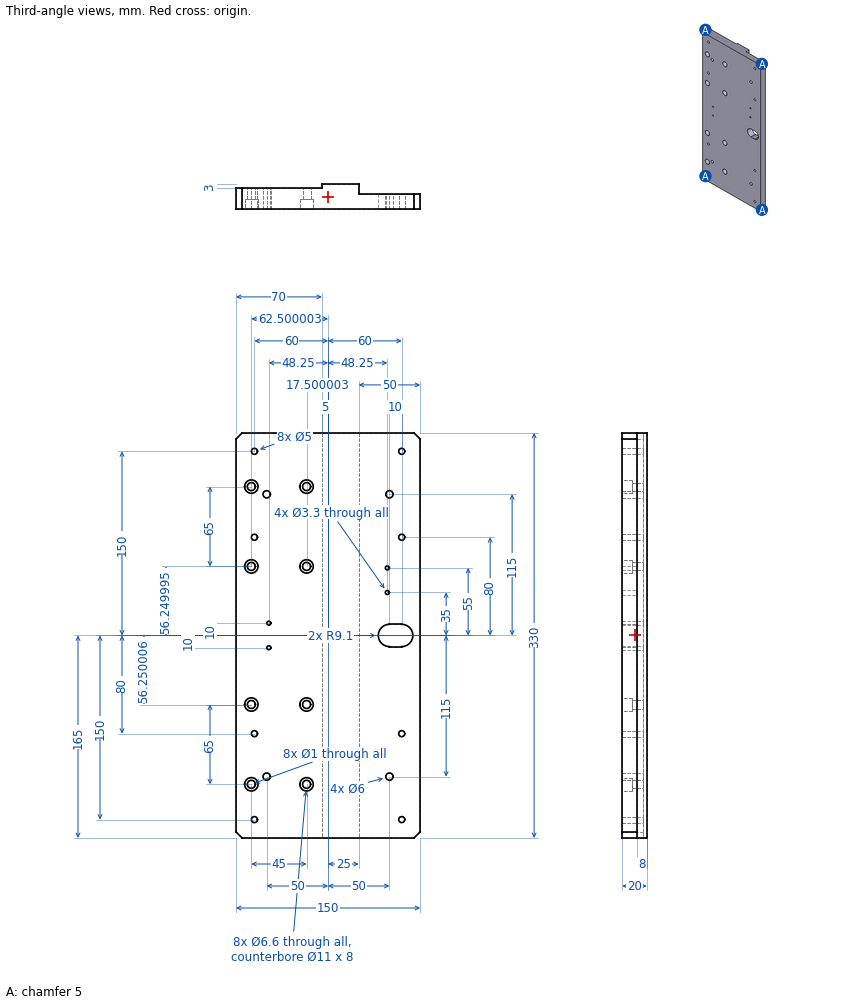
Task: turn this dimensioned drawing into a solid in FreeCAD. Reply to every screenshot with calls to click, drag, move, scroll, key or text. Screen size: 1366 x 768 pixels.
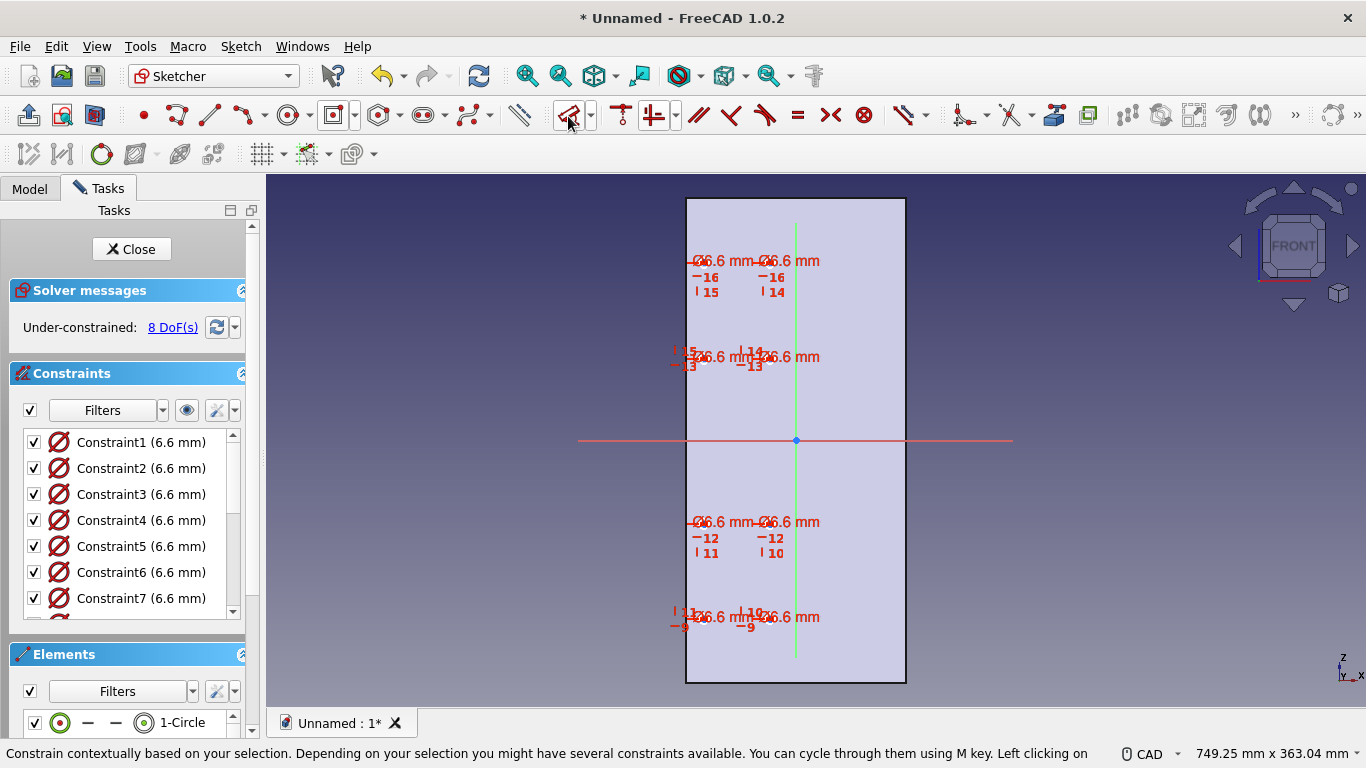
click(770, 619)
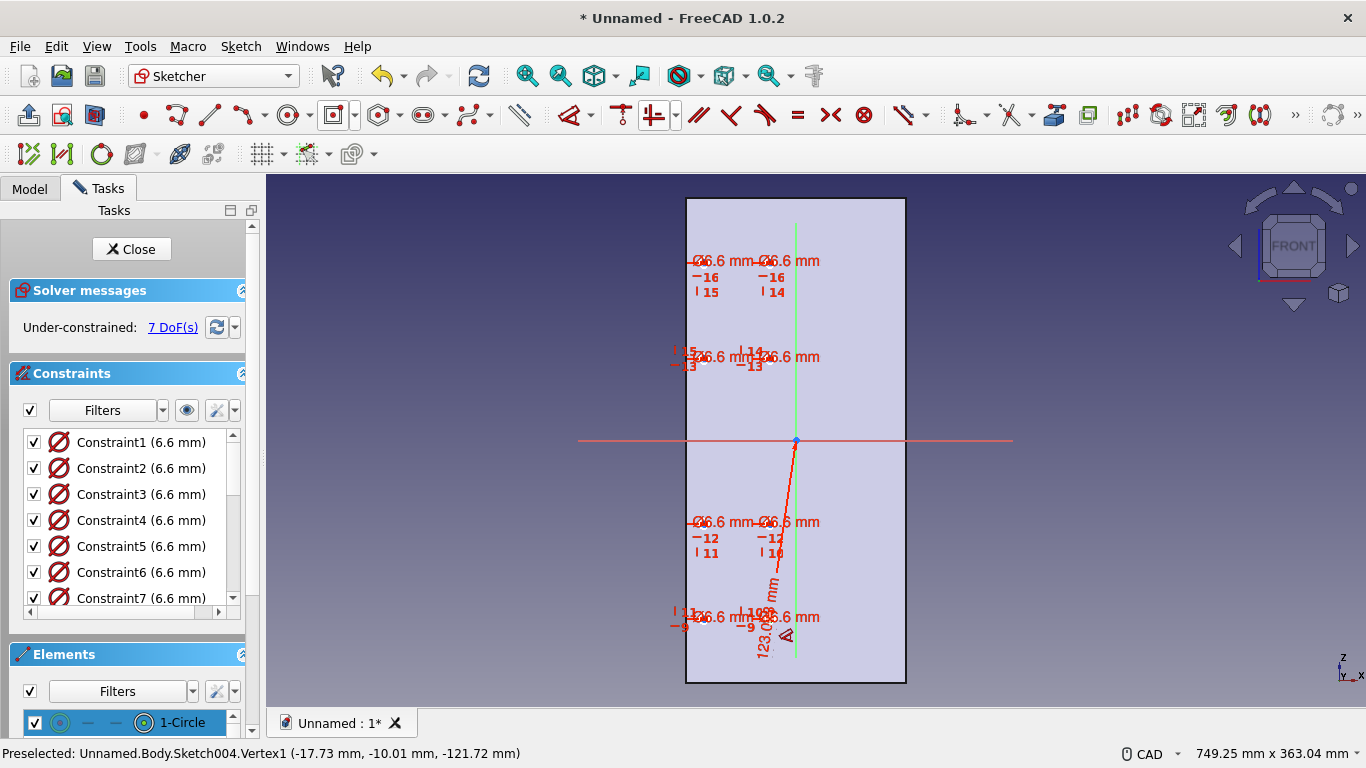
click(704, 619)
click(737, 653)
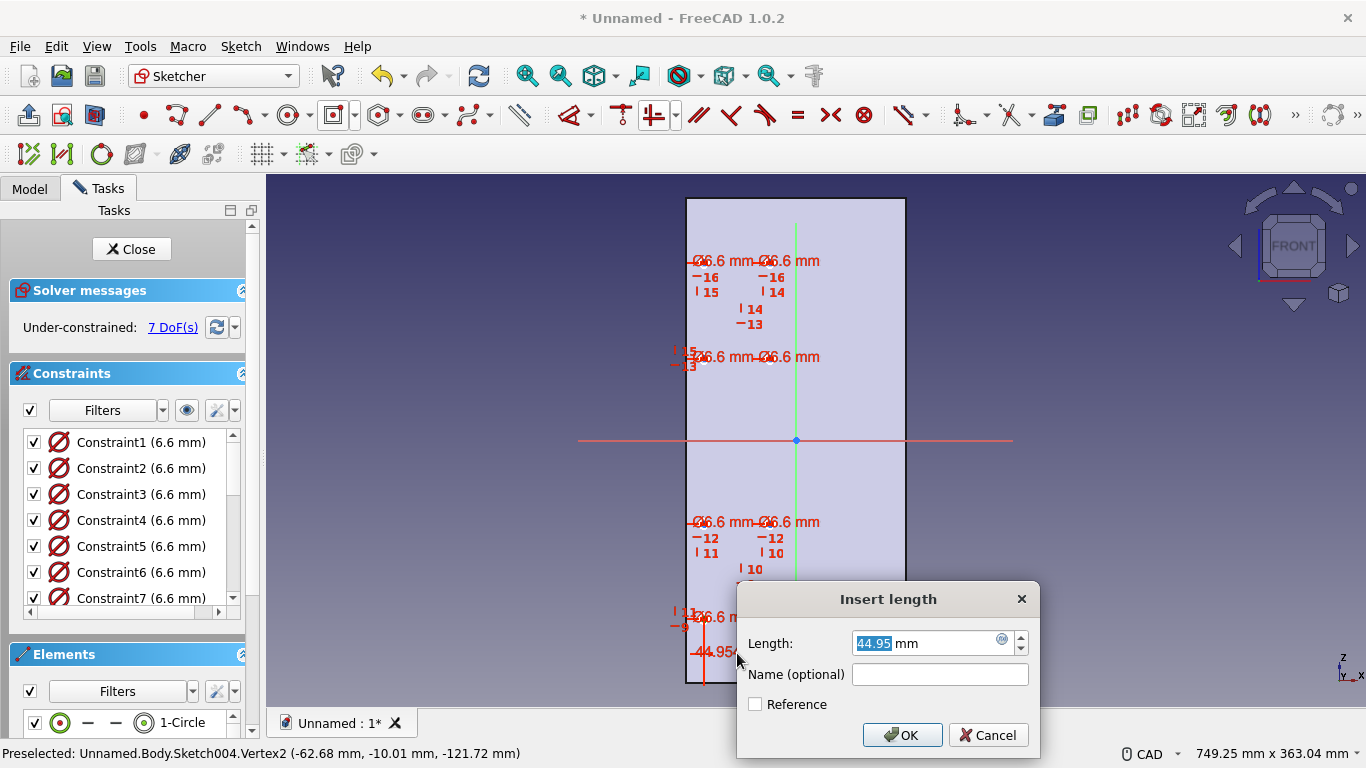
text(45)
key(Return)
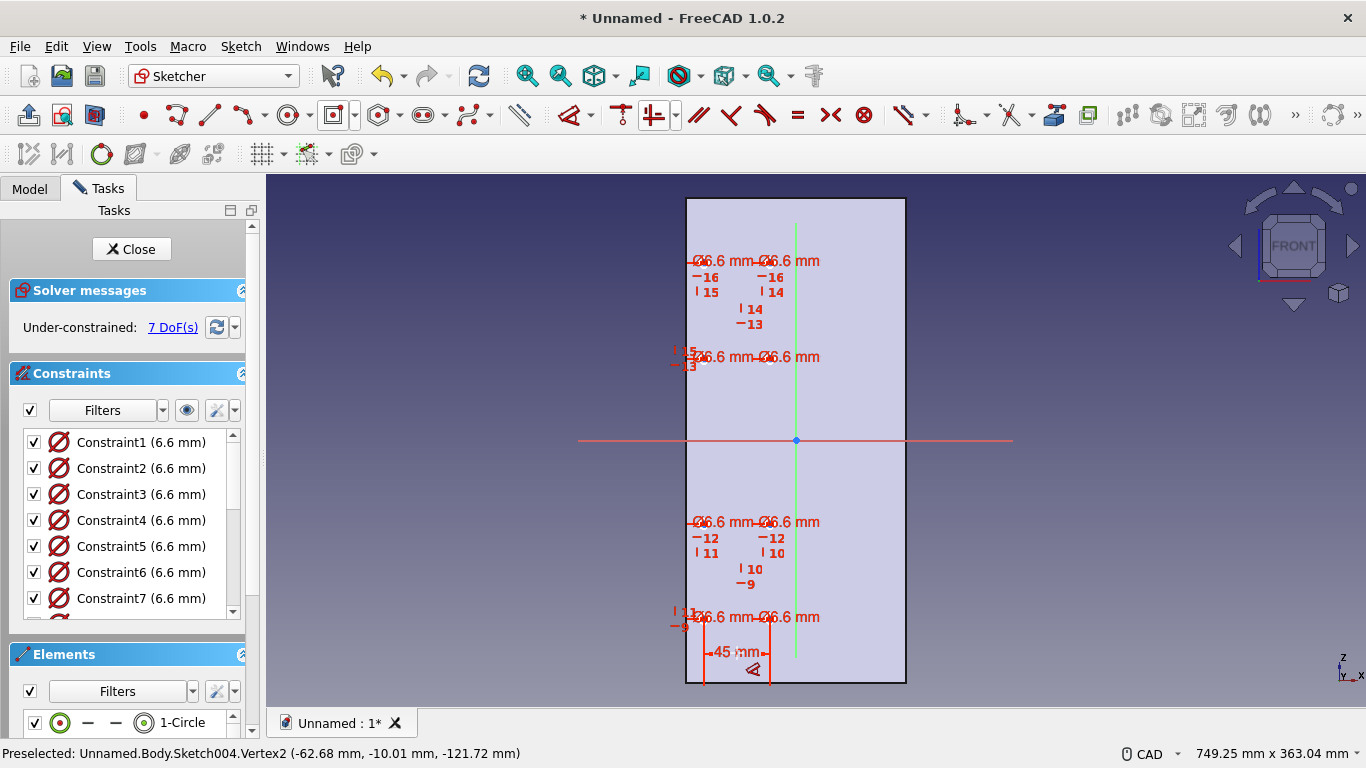
click(770, 619)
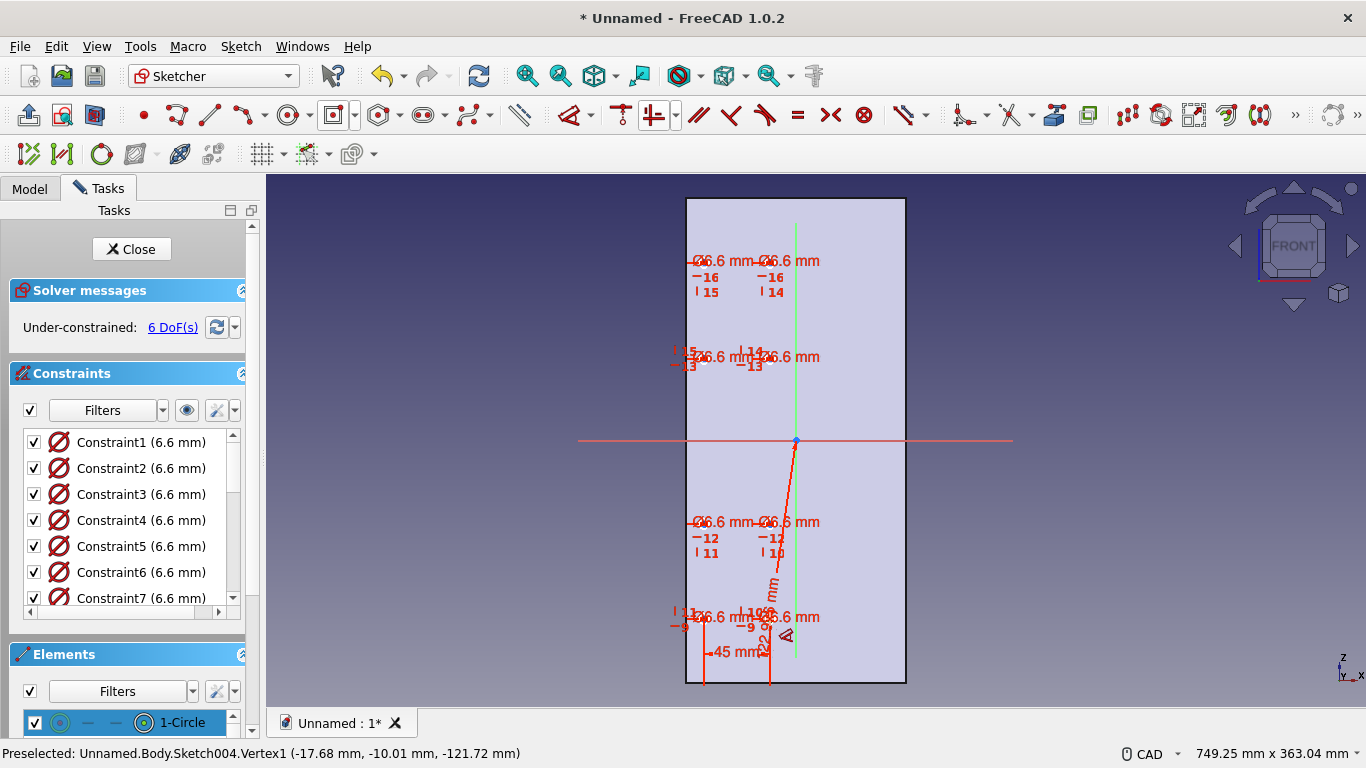
click(770, 524)
click(736, 572)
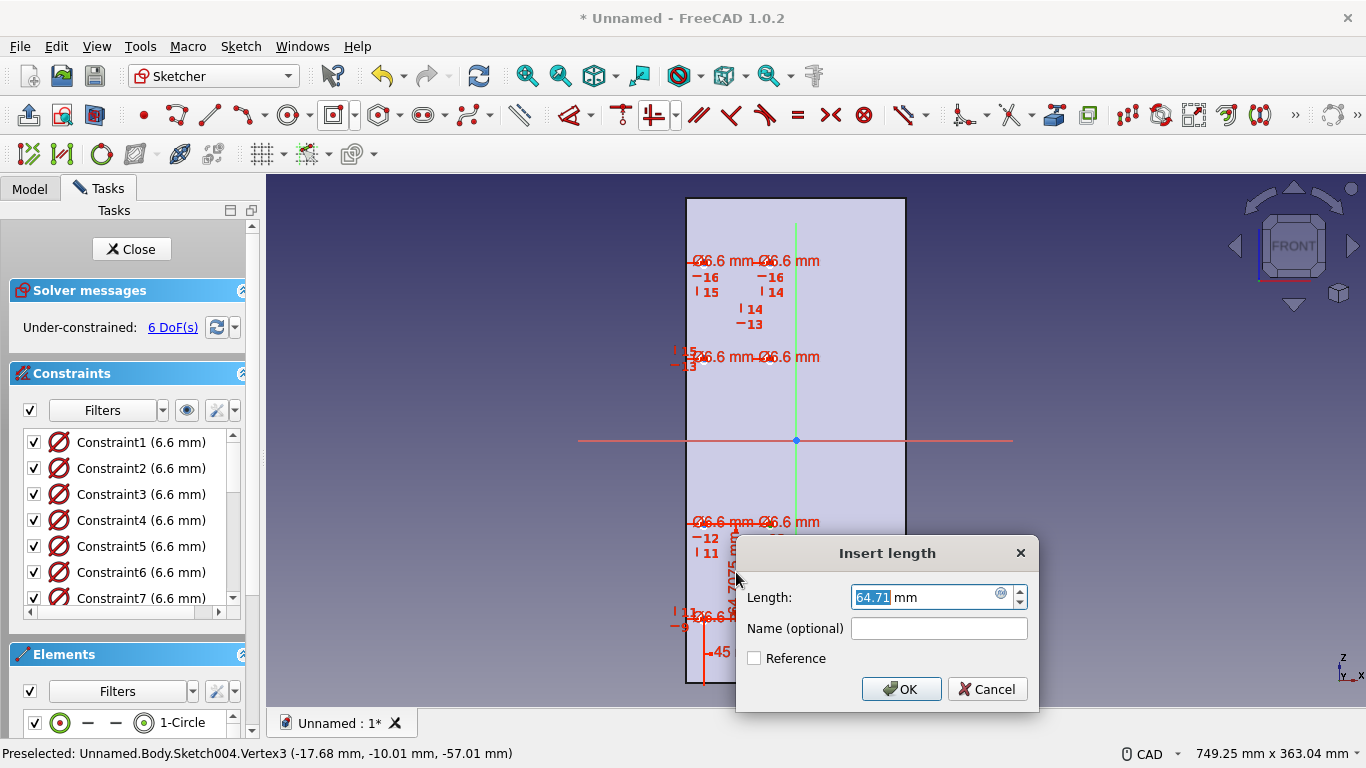
text(65)
key(Return)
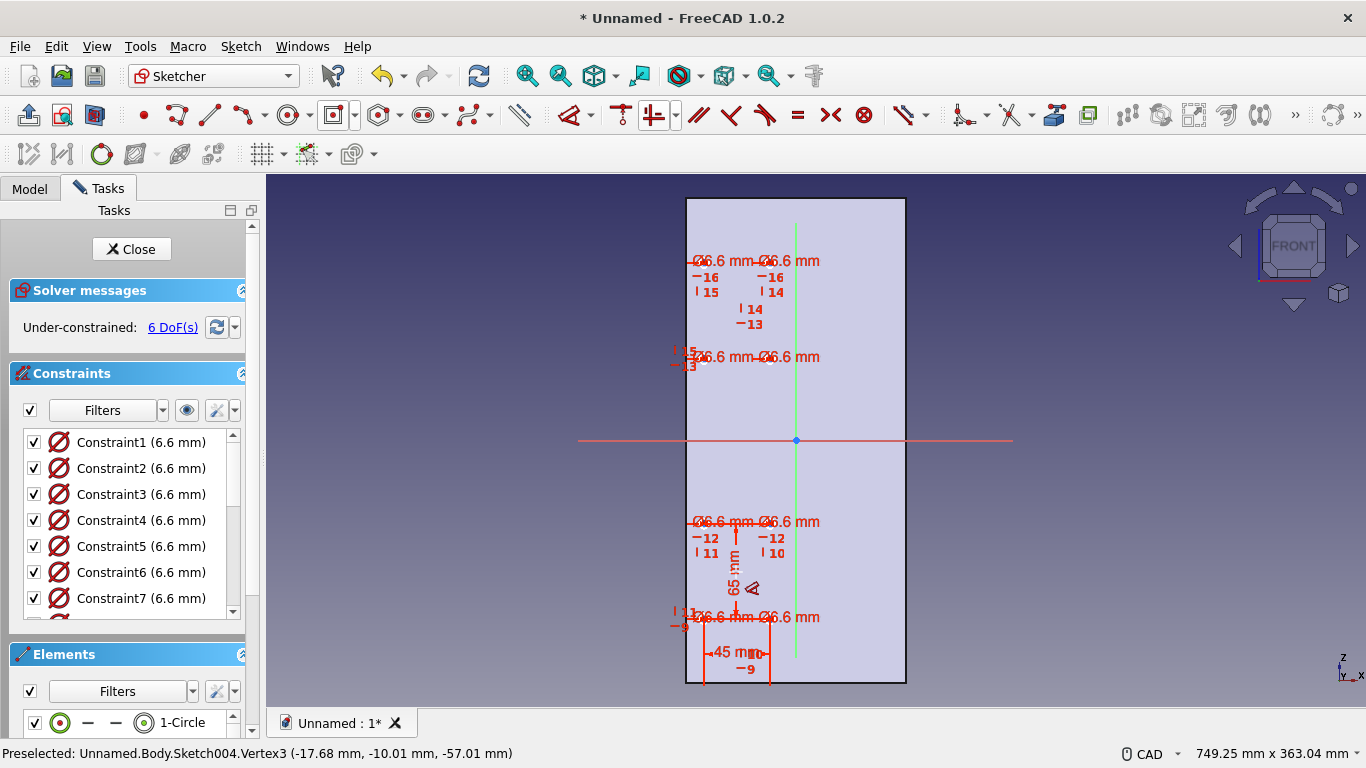
click(770, 359)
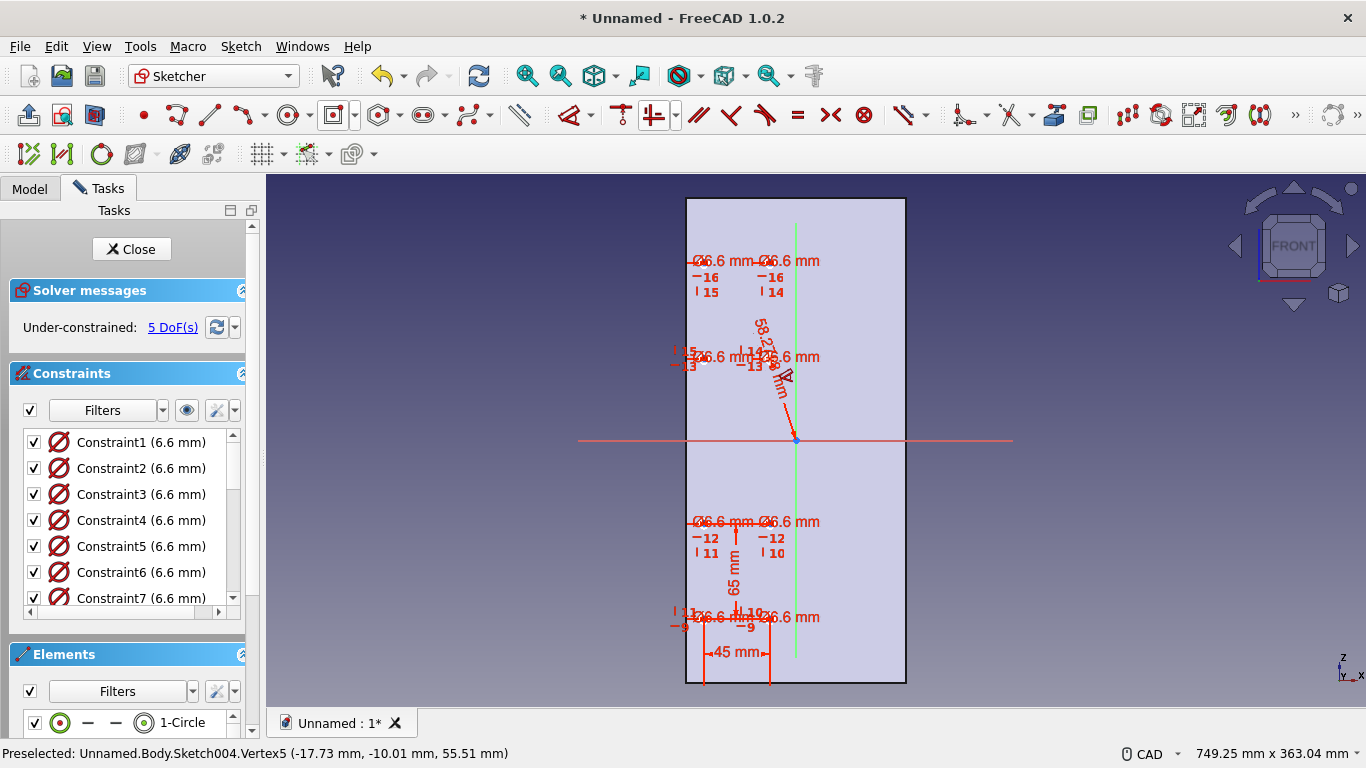
click(704, 359)
click(737, 325)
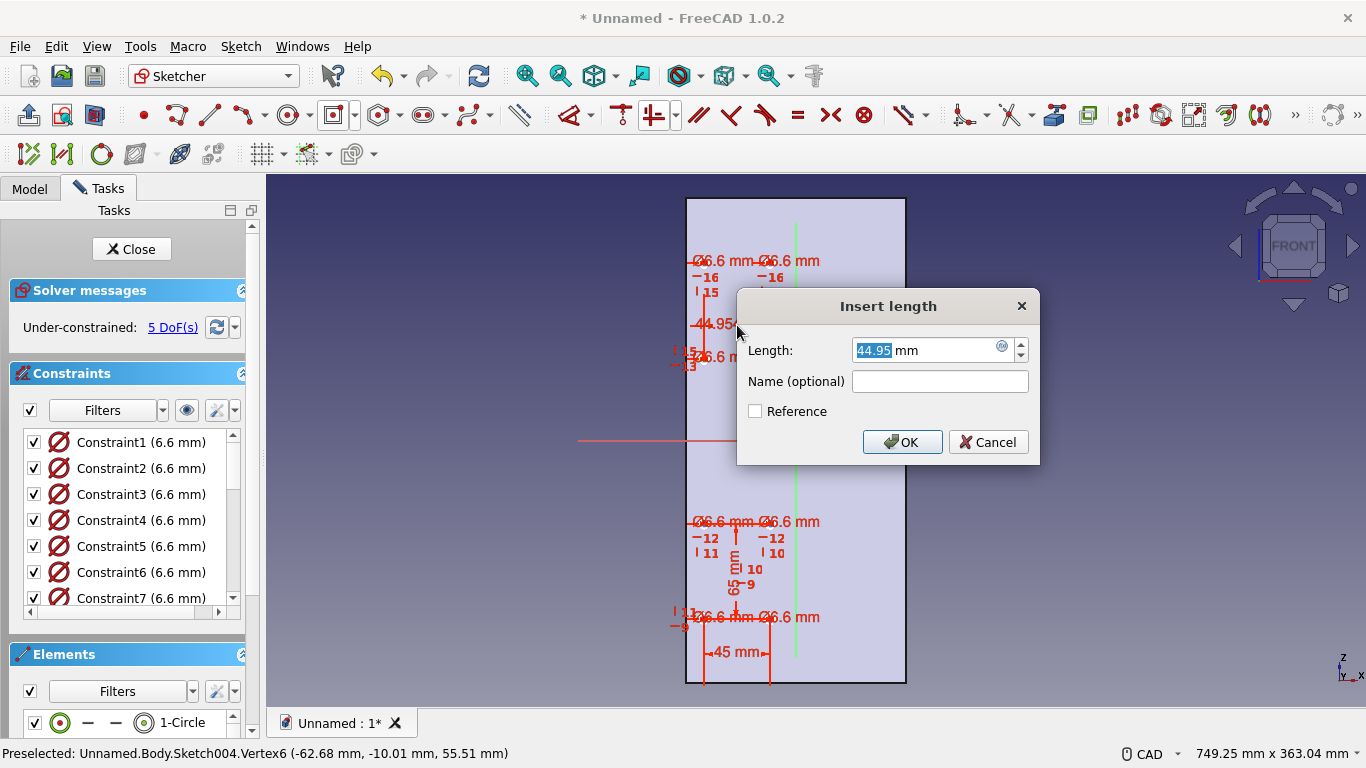
text(45)
key(Return)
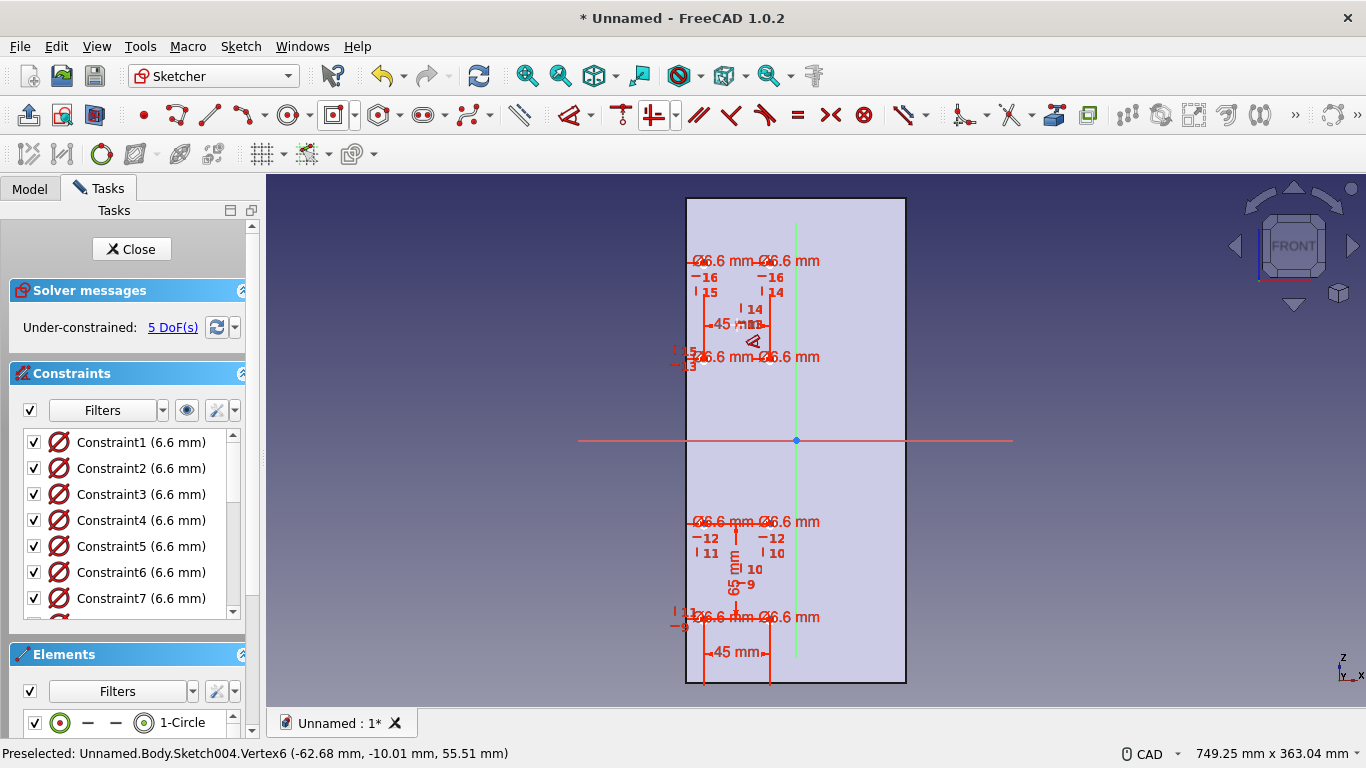
click(770, 359)